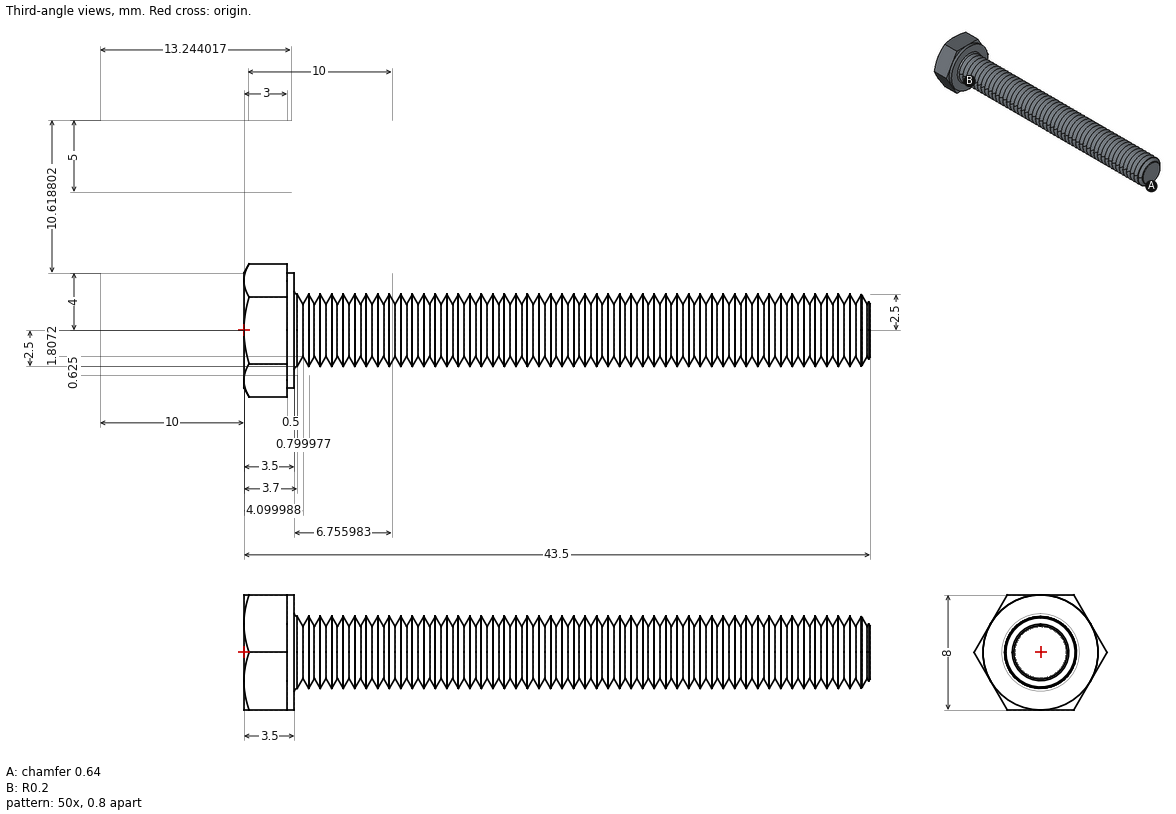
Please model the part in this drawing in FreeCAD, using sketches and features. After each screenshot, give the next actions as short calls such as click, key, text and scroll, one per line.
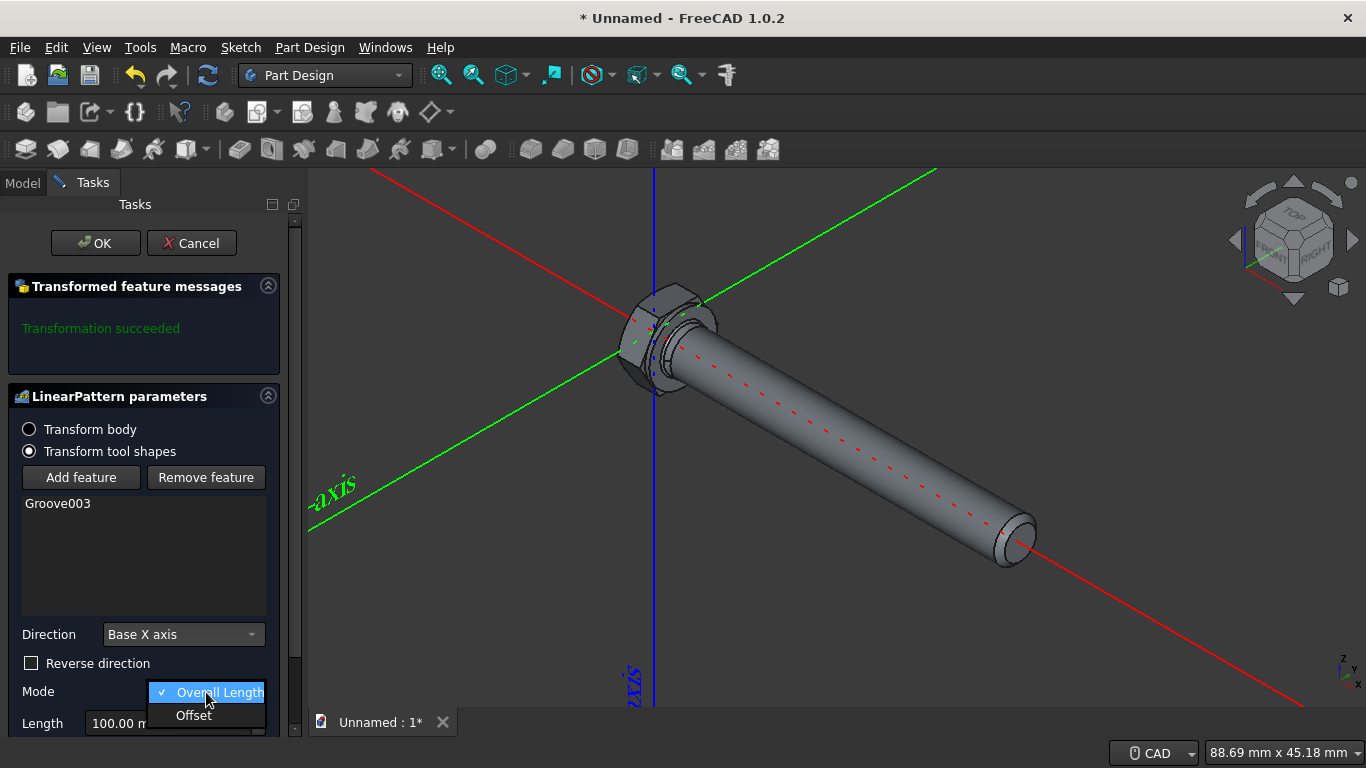
click(206, 716)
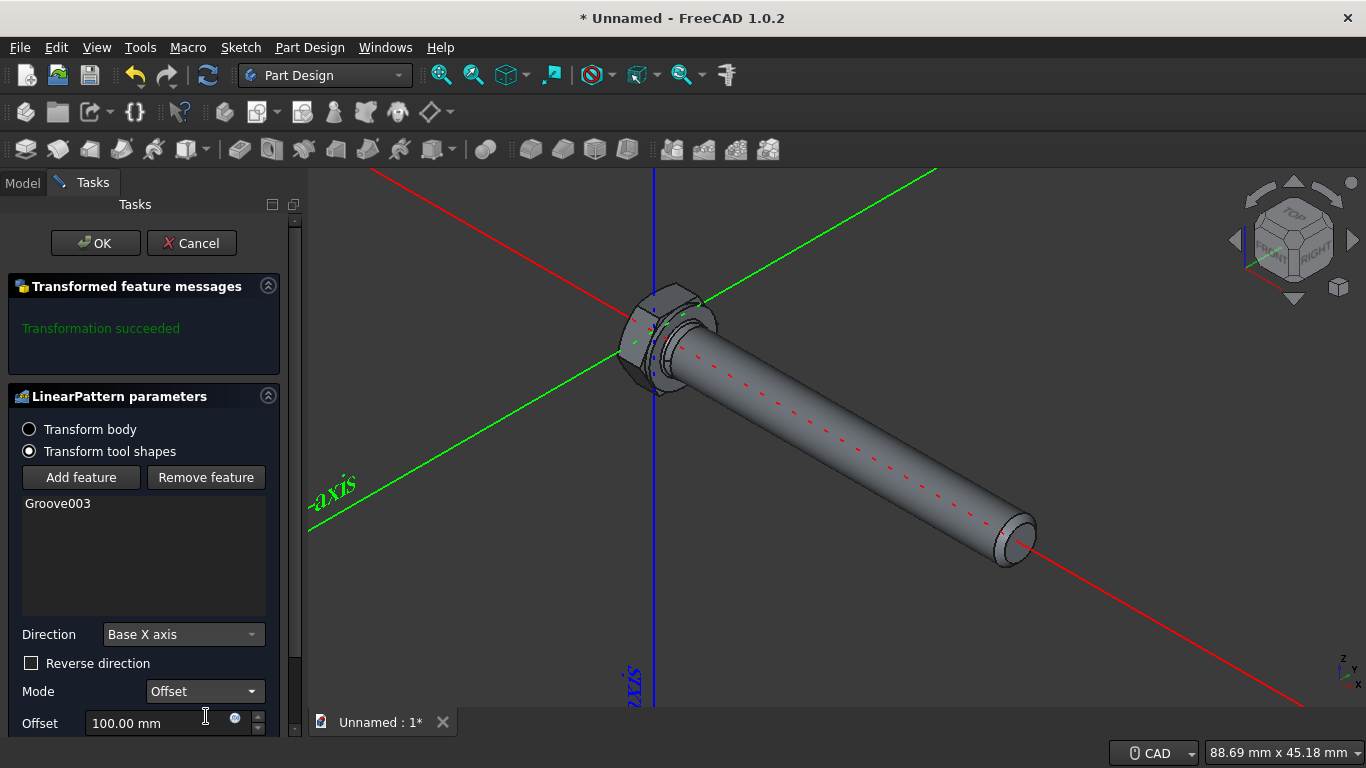
triple_click(168, 723)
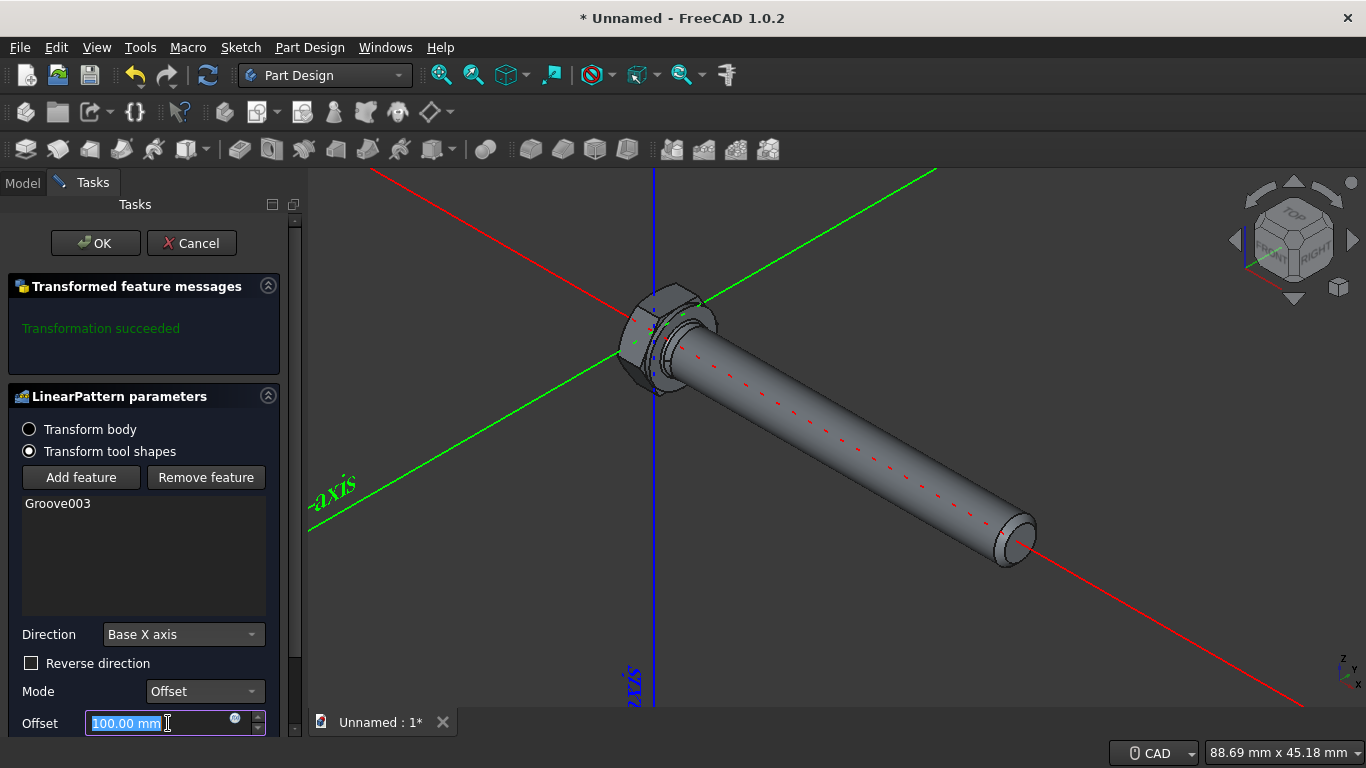
text(0.8)
key(Tab)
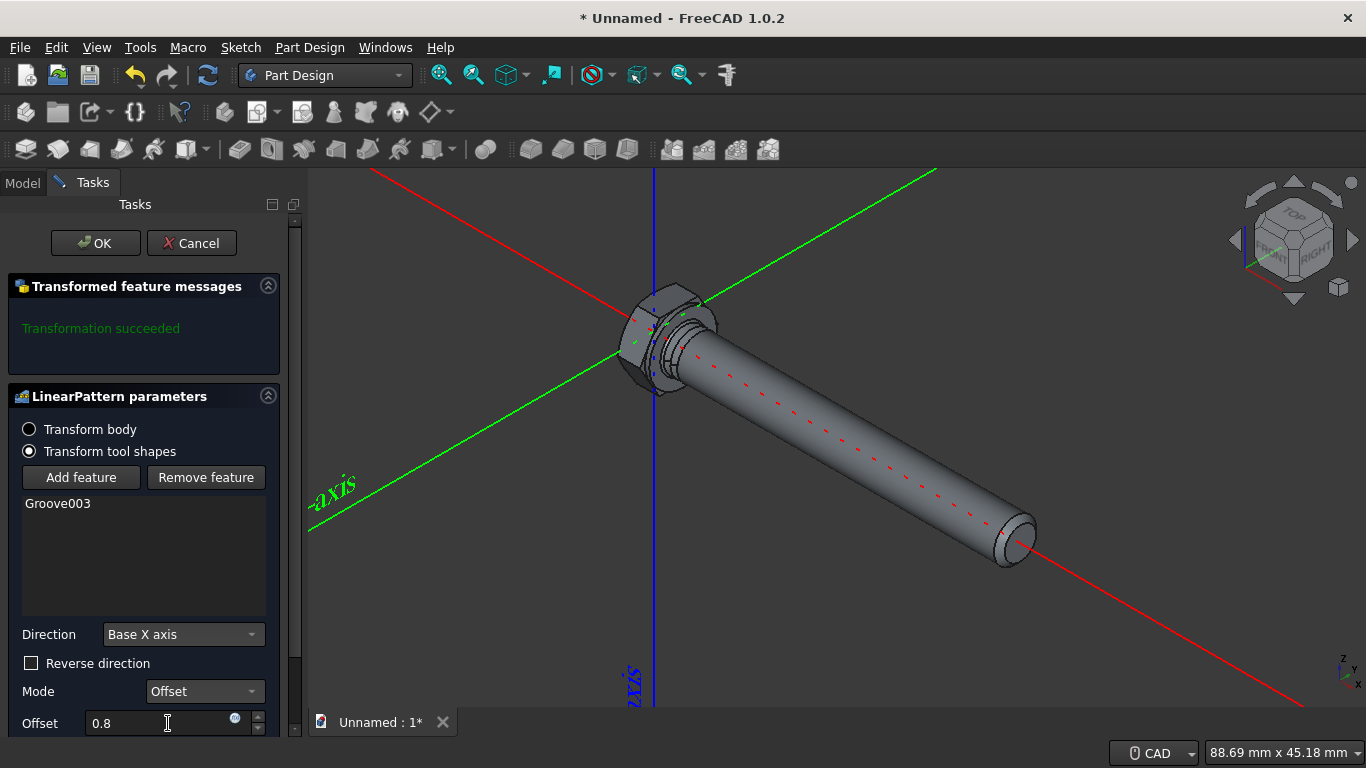
scroll(295, 475, down, 2)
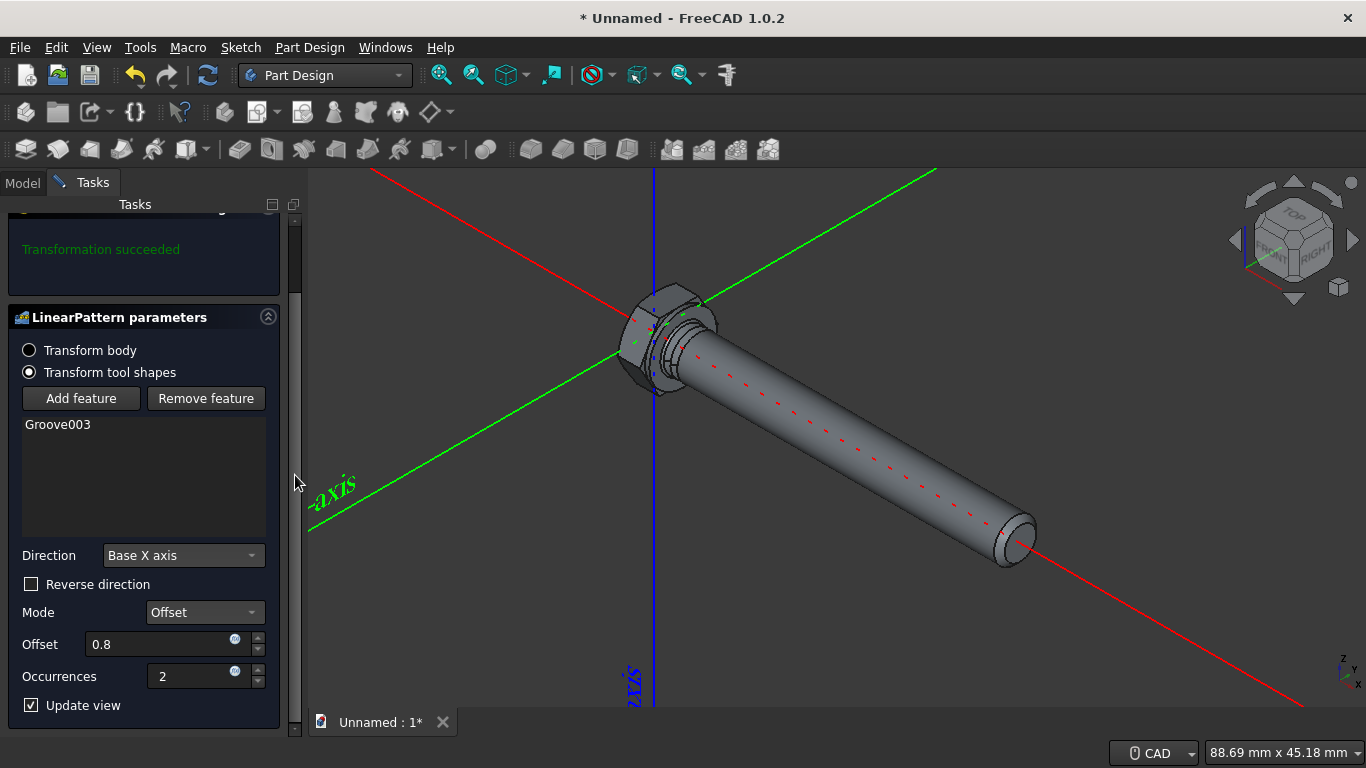
triple_click(198, 676)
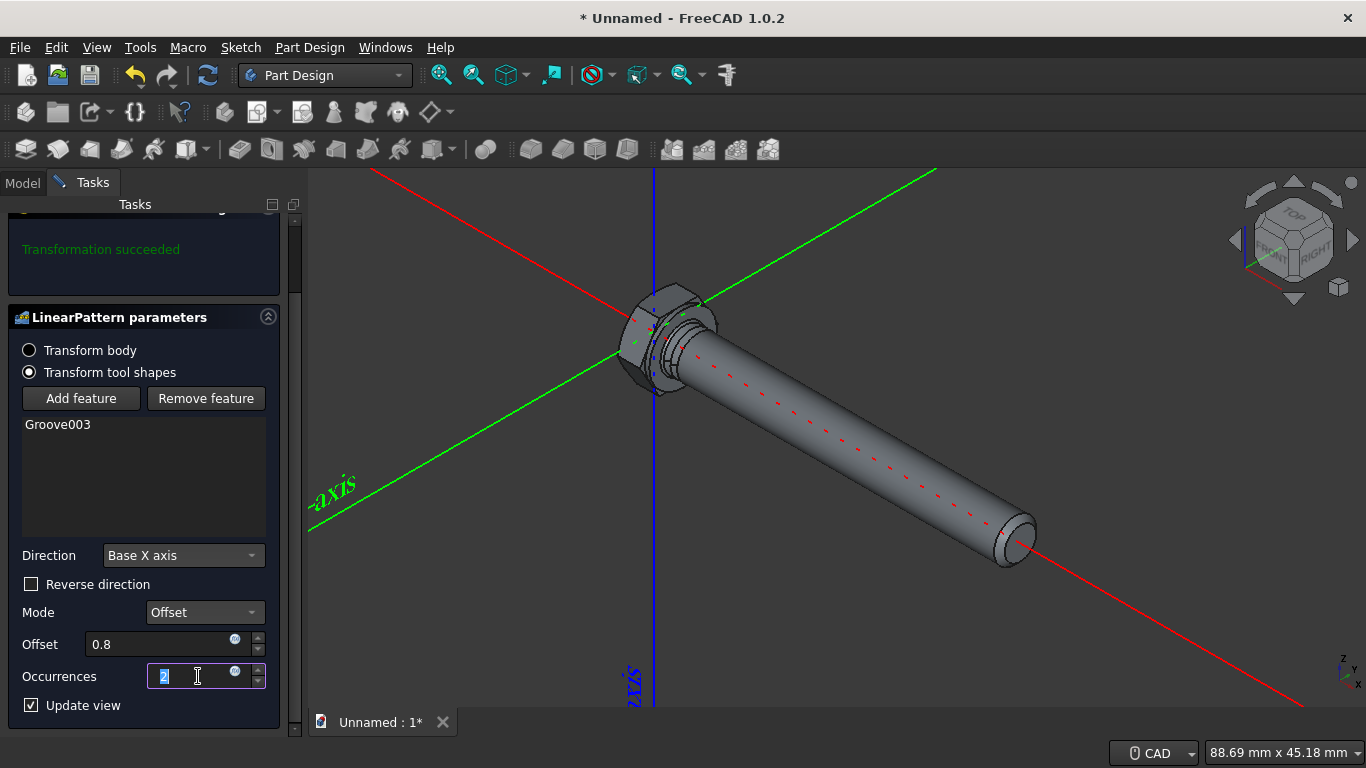
text(50)
key(Tab)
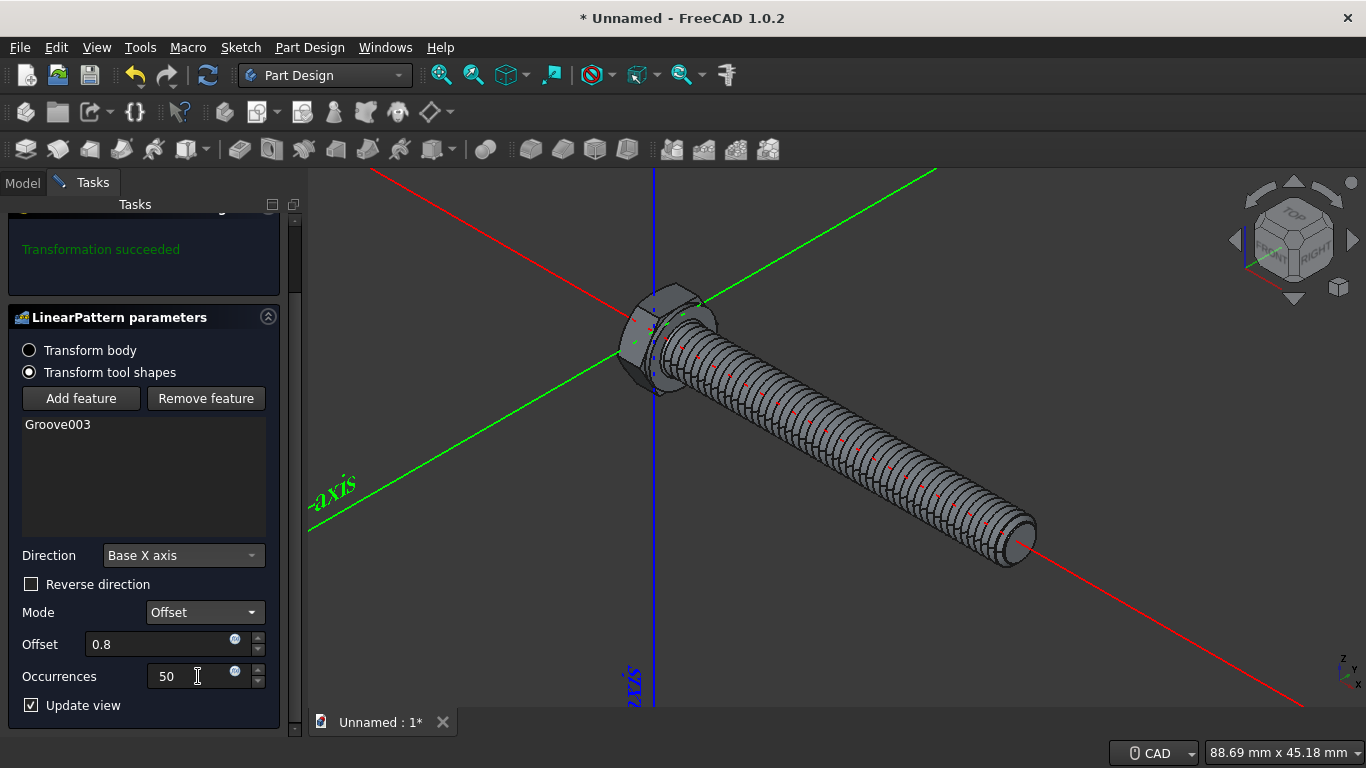
scroll(295, 475, up, 3)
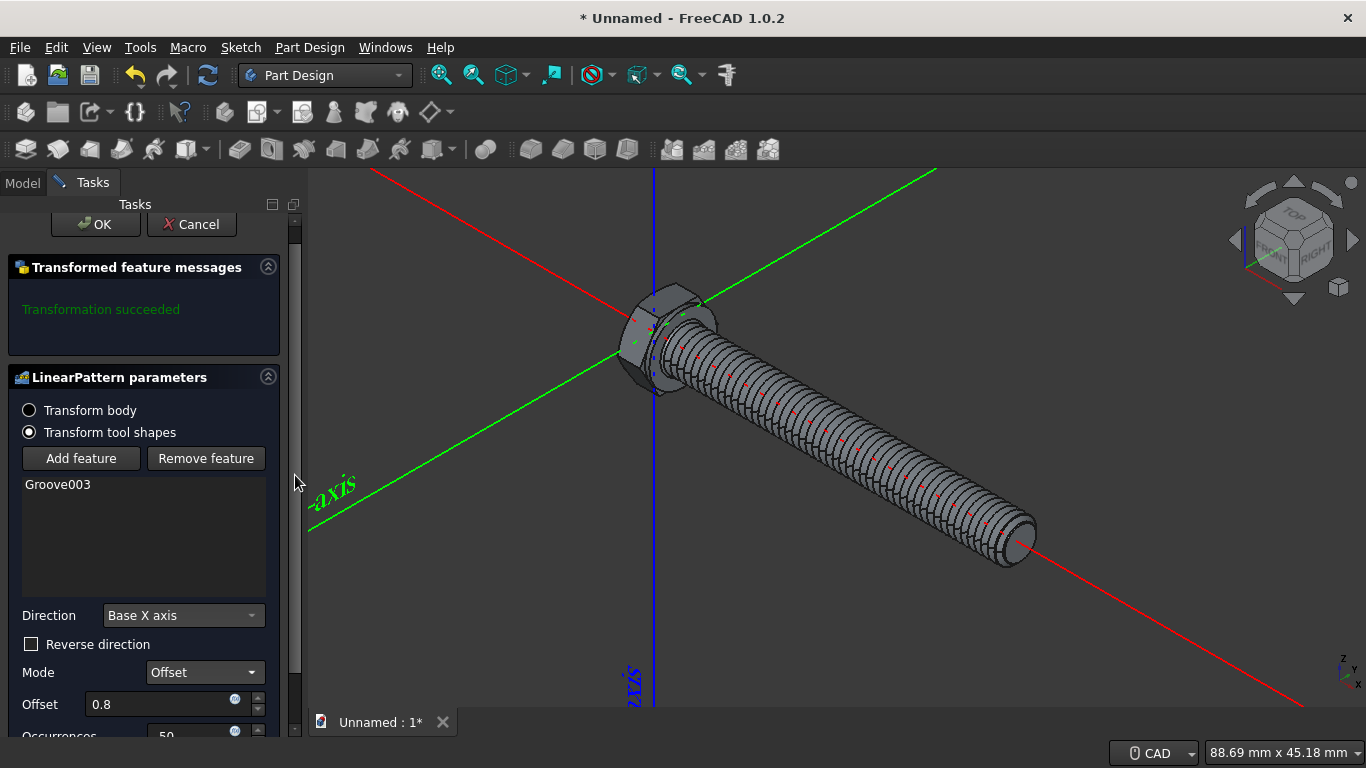
click(96, 243)